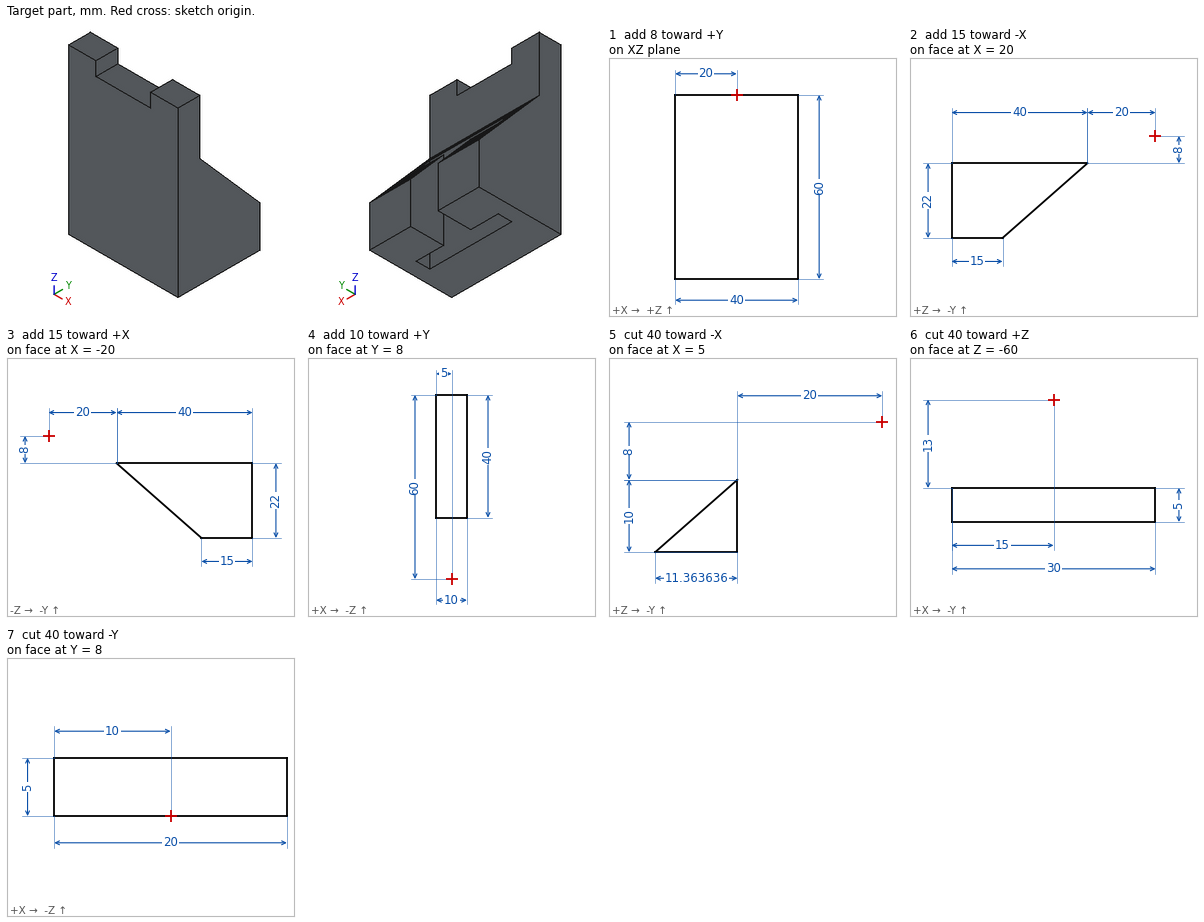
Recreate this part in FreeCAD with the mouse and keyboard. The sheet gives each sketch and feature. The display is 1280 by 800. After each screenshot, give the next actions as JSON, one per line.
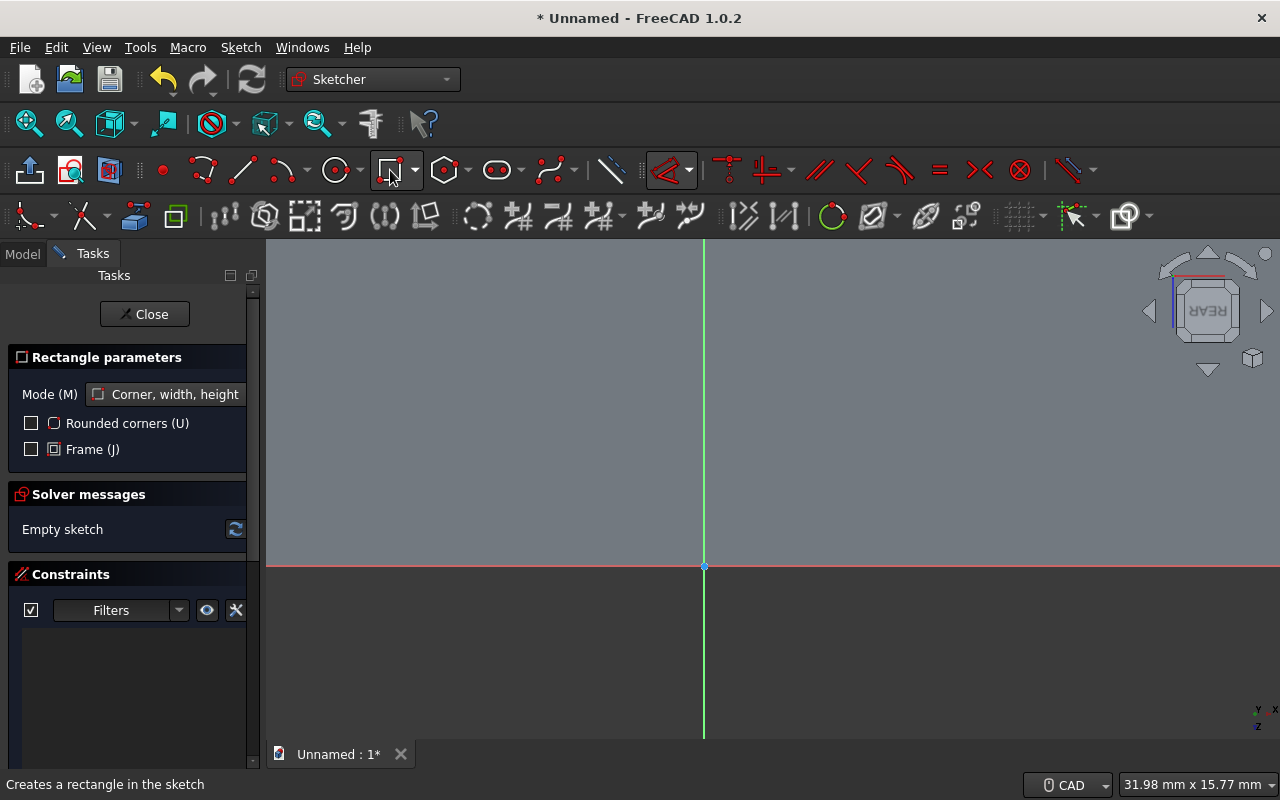
{"action": "left_click", "coordinate": [387, 408]}
{"action": "left_click", "coordinate": [1021, 566]}
{"action": "key", "text": "Escape"}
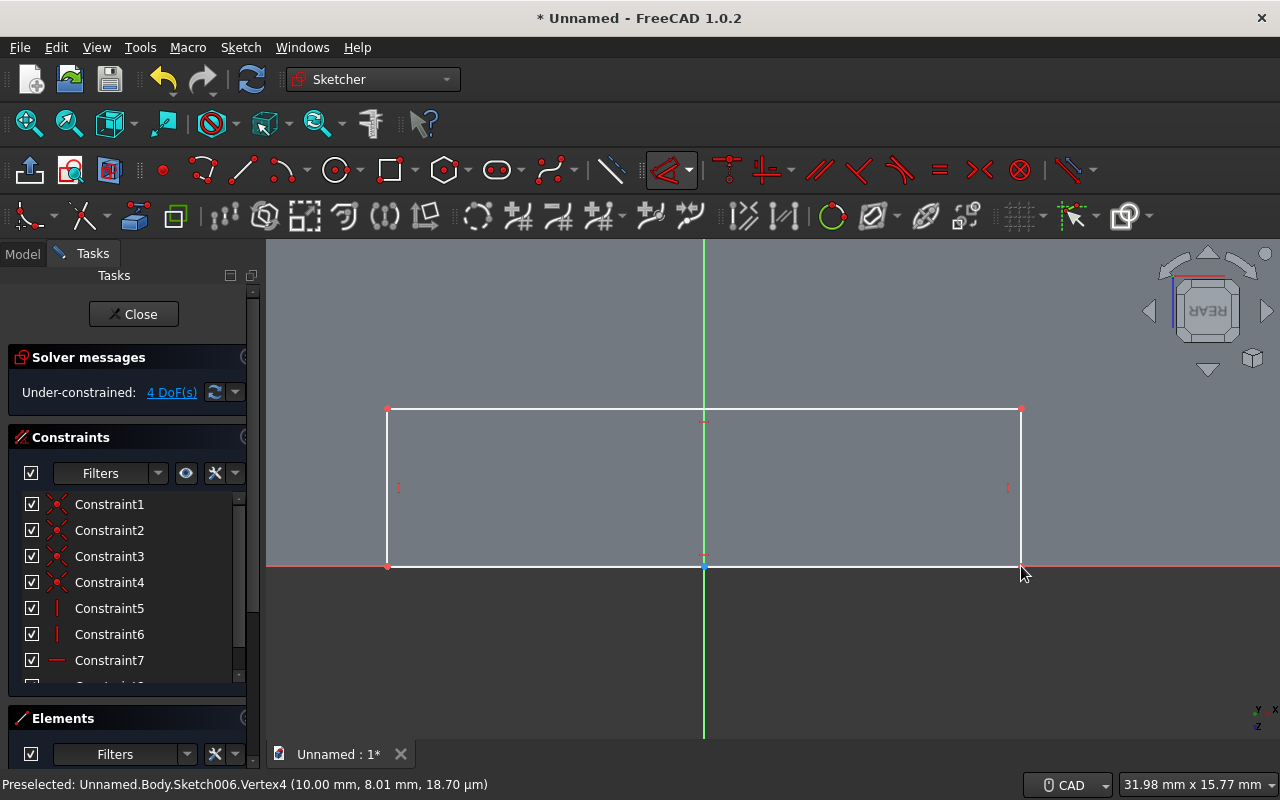
{"action": "left_click", "coordinate": [387, 567]}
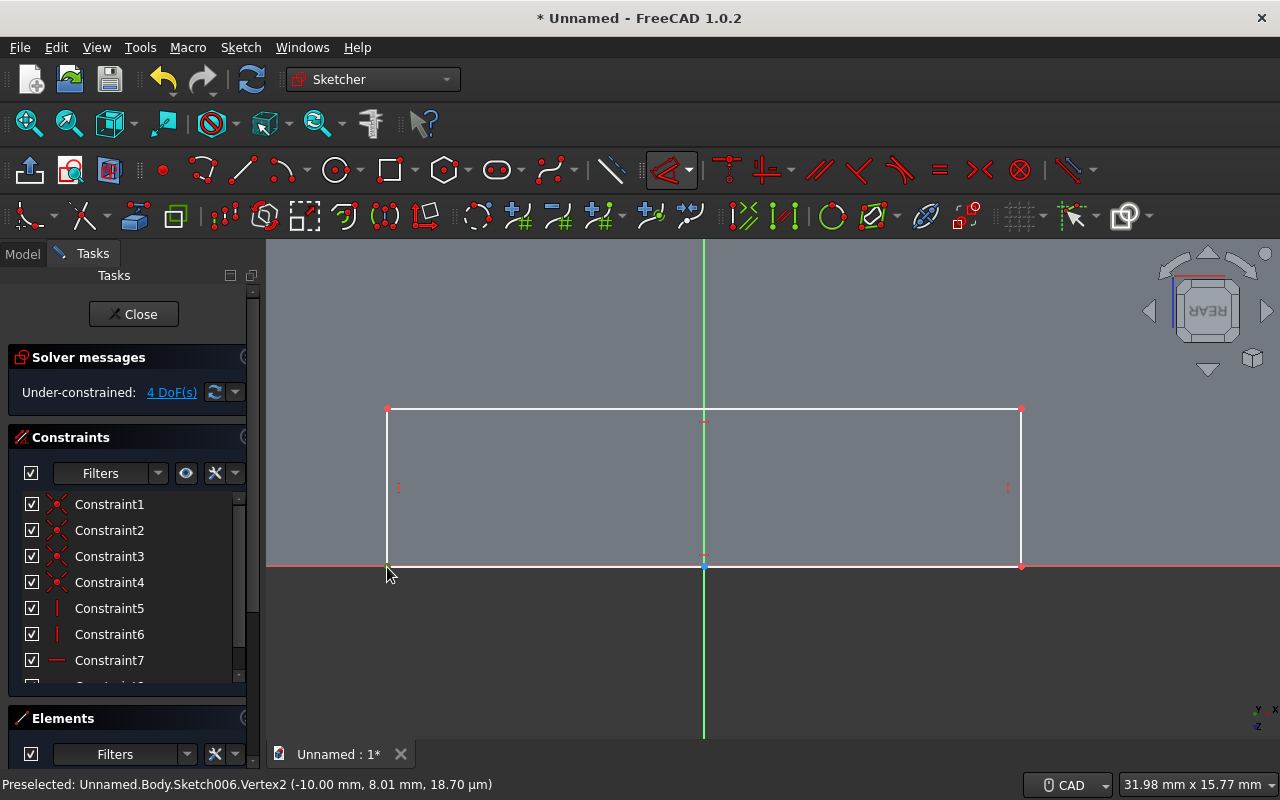
{"action": "left_click", "coordinate": [353, 566]}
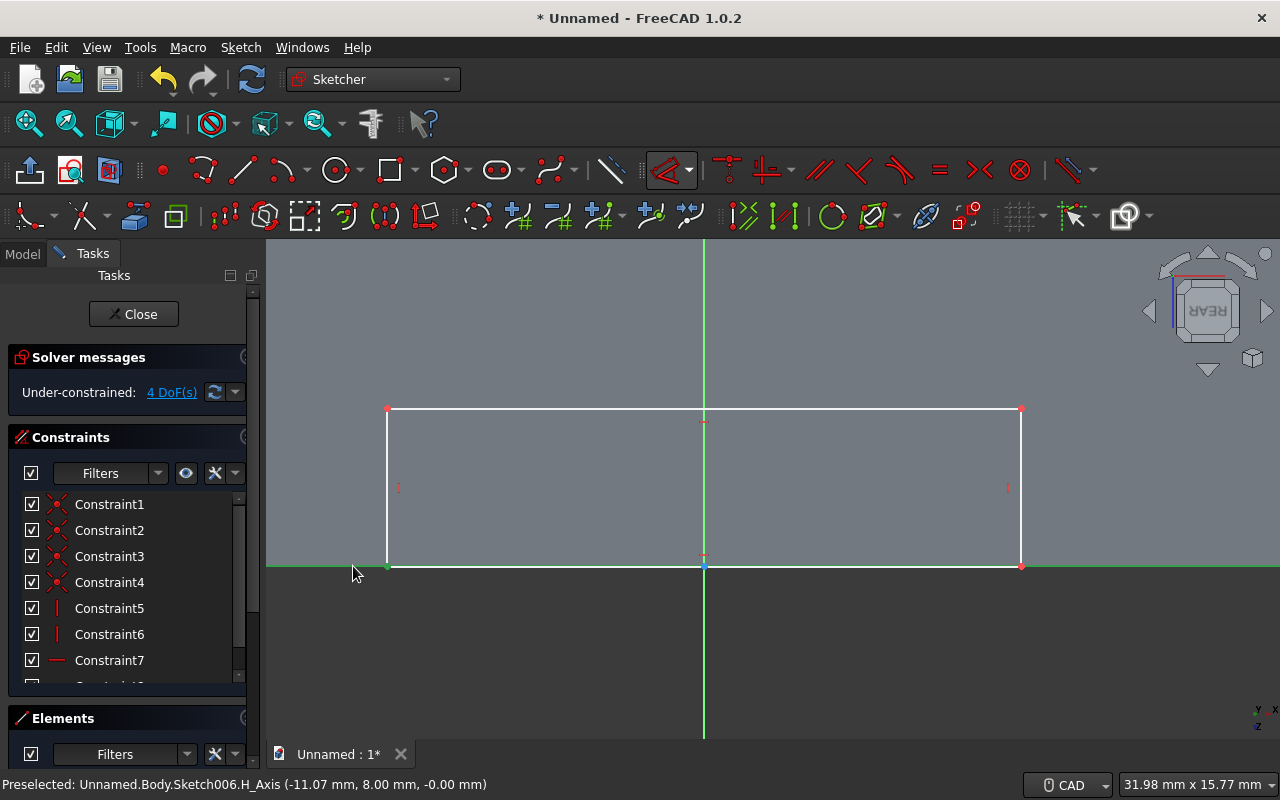
{"action": "left_click", "coordinate": [728, 170]}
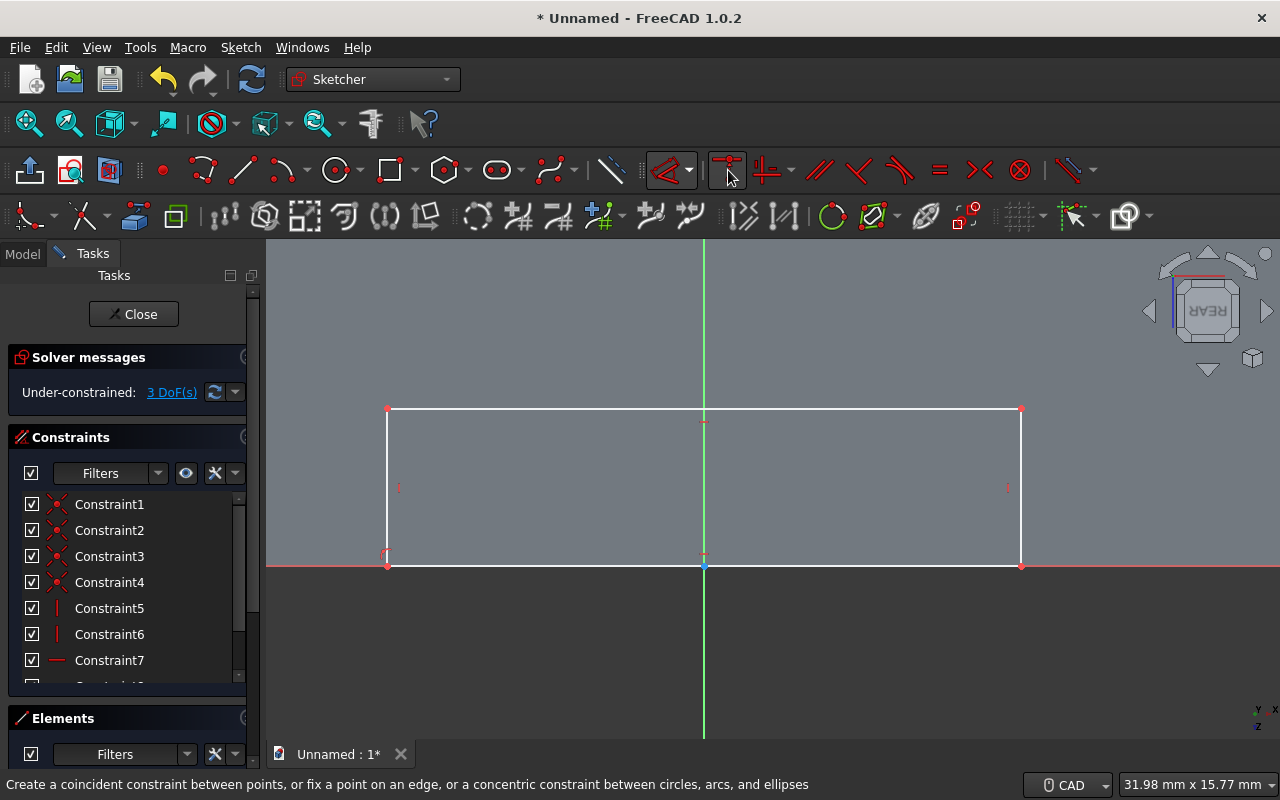
{"action": "left_click", "coordinate": [387, 456]}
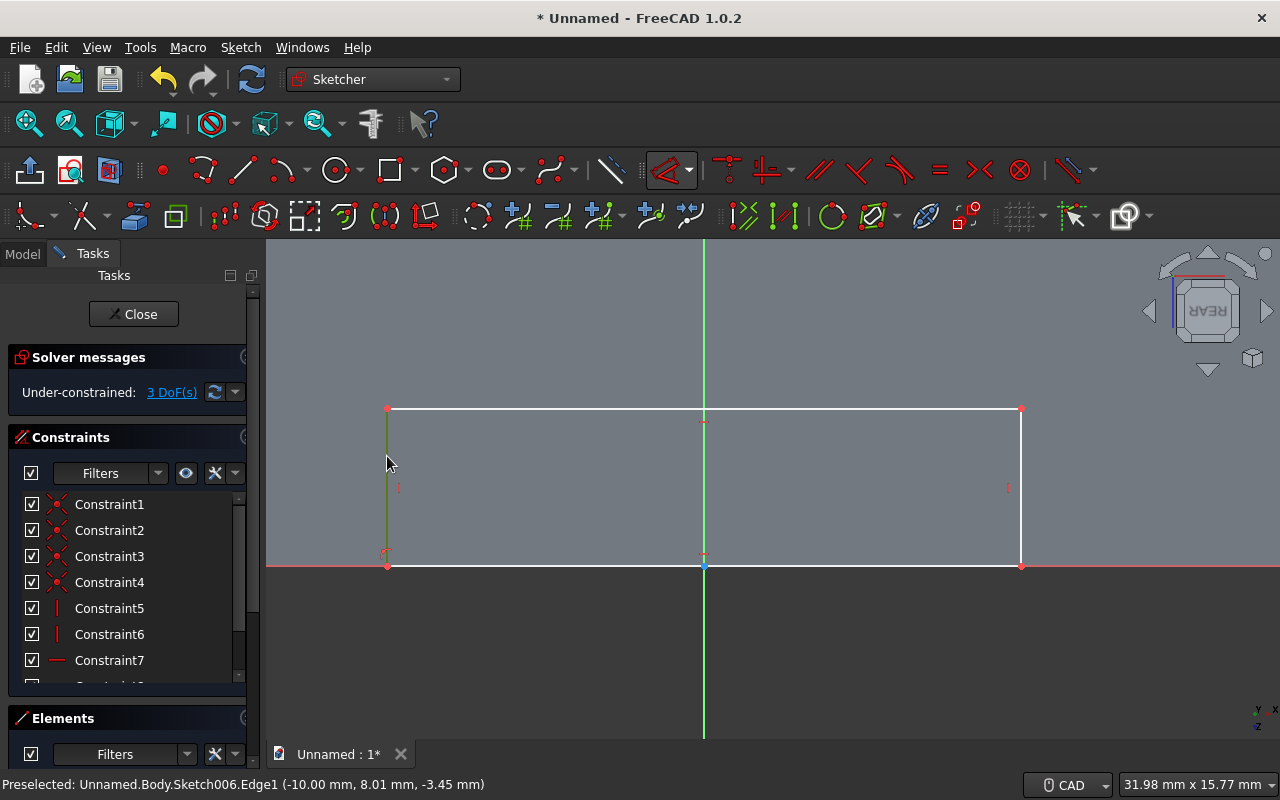
{"action": "key", "text": "i"}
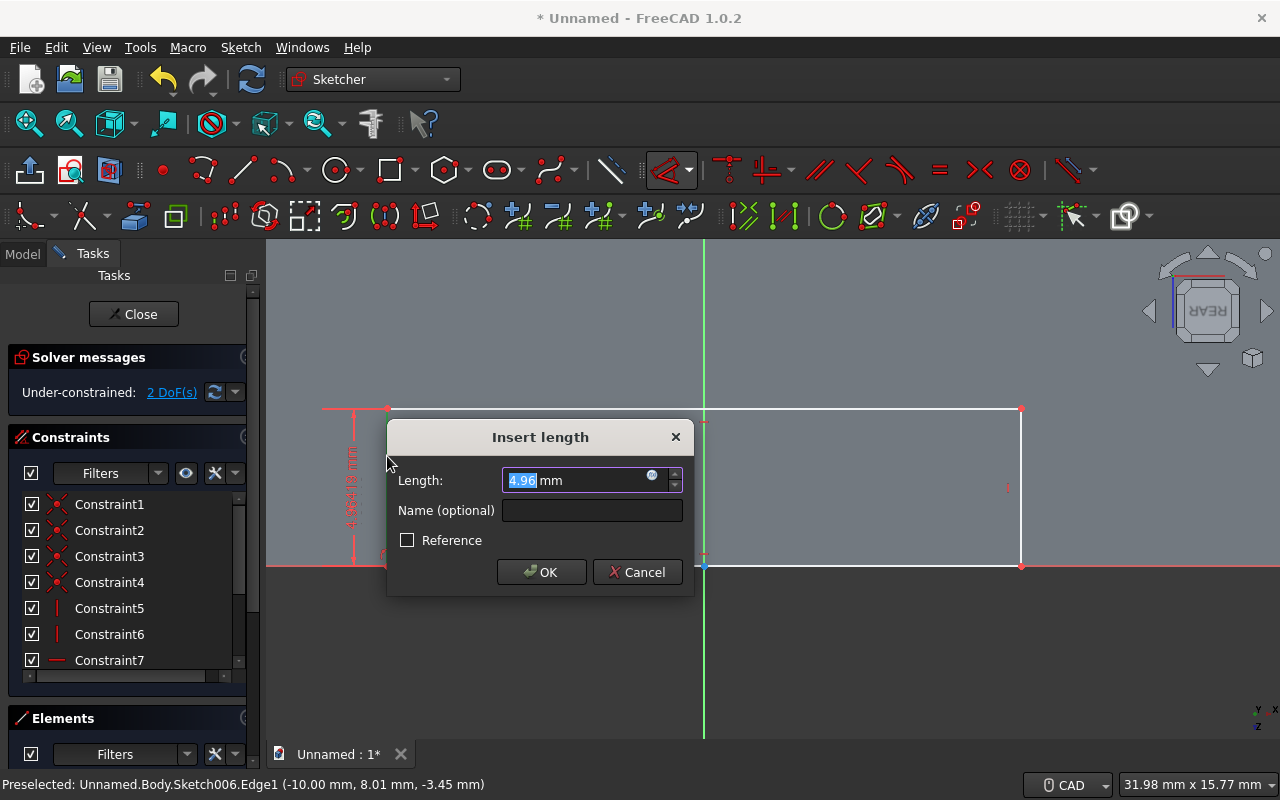
{"action": "type", "text": "5"}
{"action": "key", "text": "Return"}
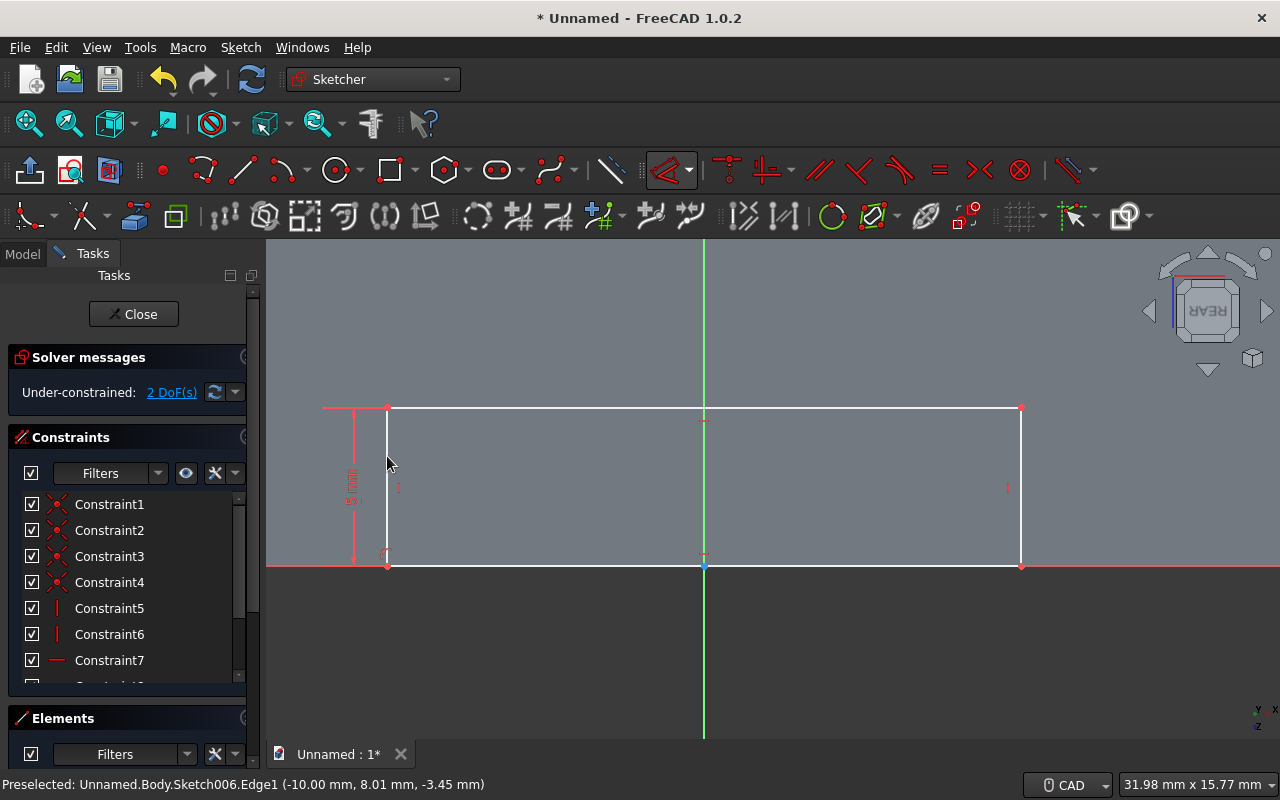
{"action": "left_click", "coordinate": [577, 566]}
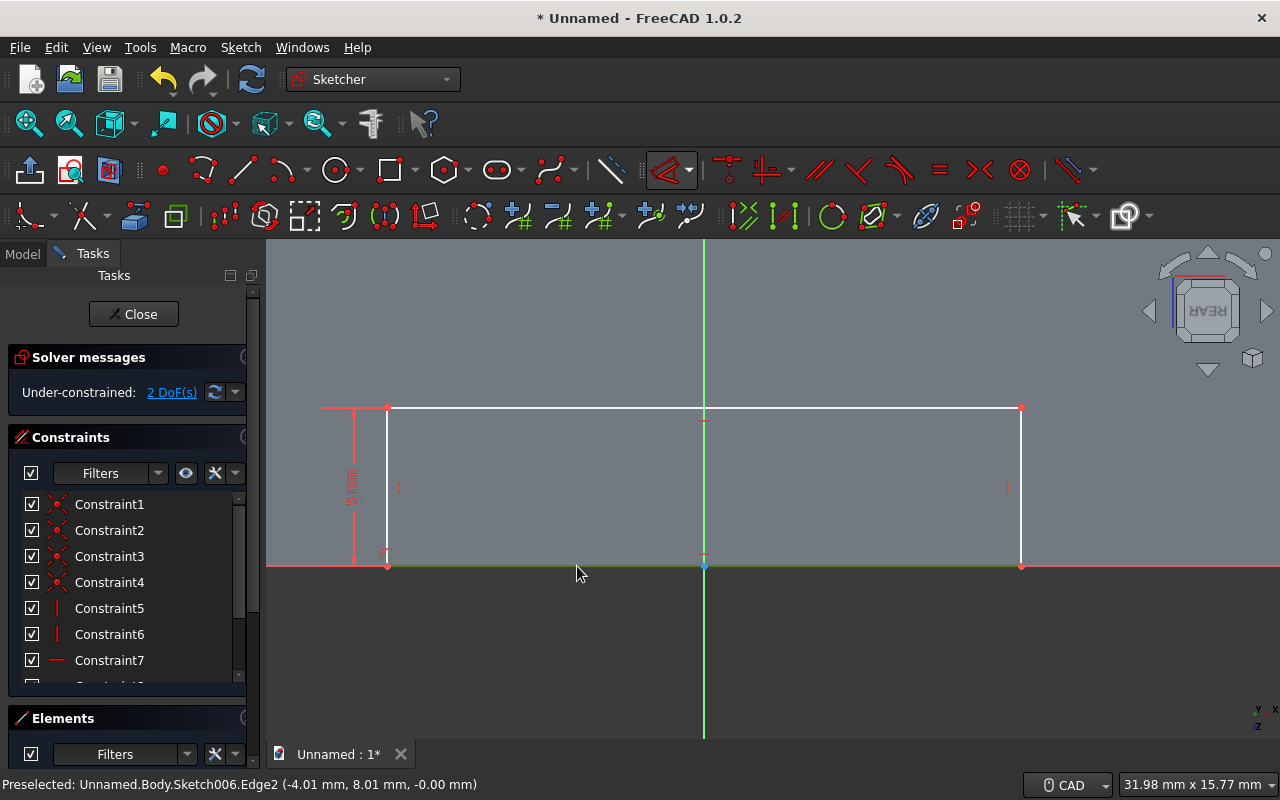
{"action": "key", "text": "l"}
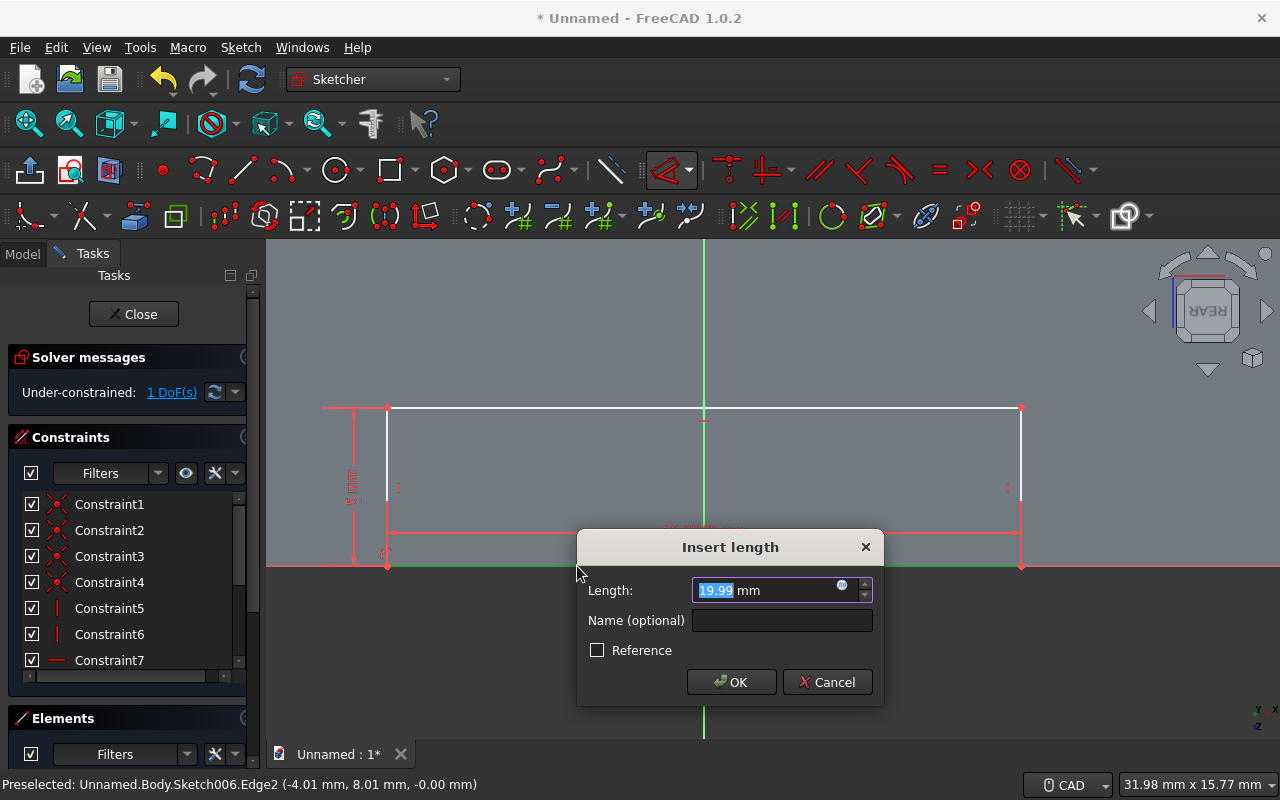
{"action": "type", "text": "20"}
{"action": "key", "text": "Return"}